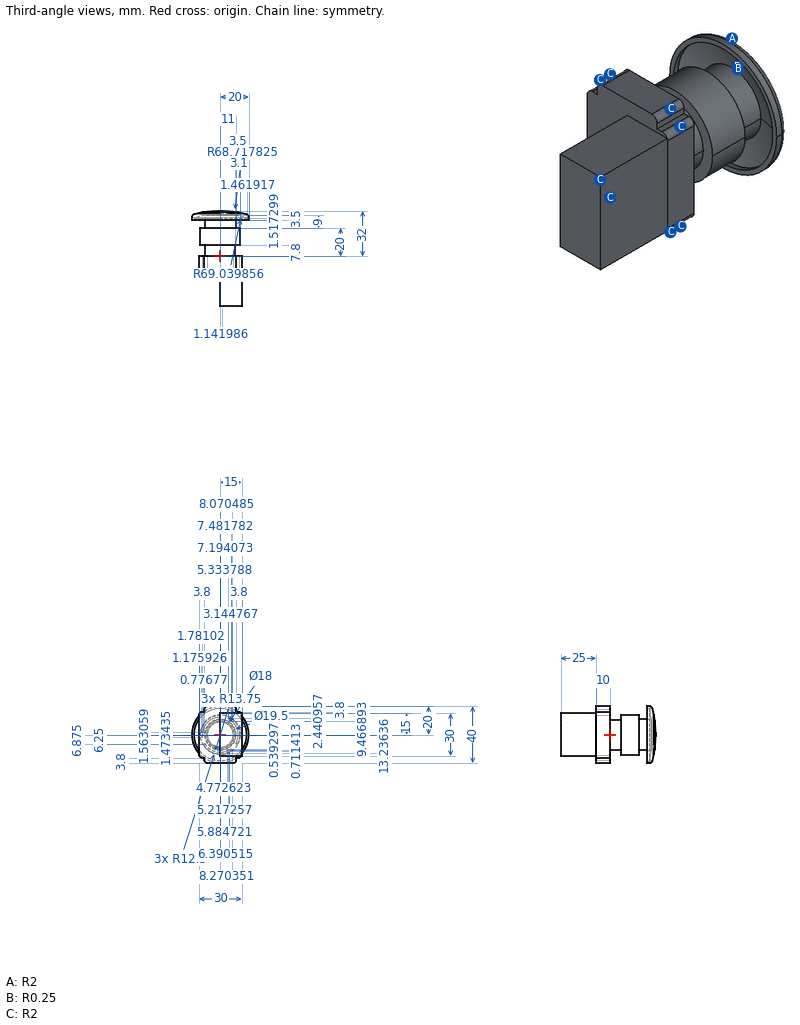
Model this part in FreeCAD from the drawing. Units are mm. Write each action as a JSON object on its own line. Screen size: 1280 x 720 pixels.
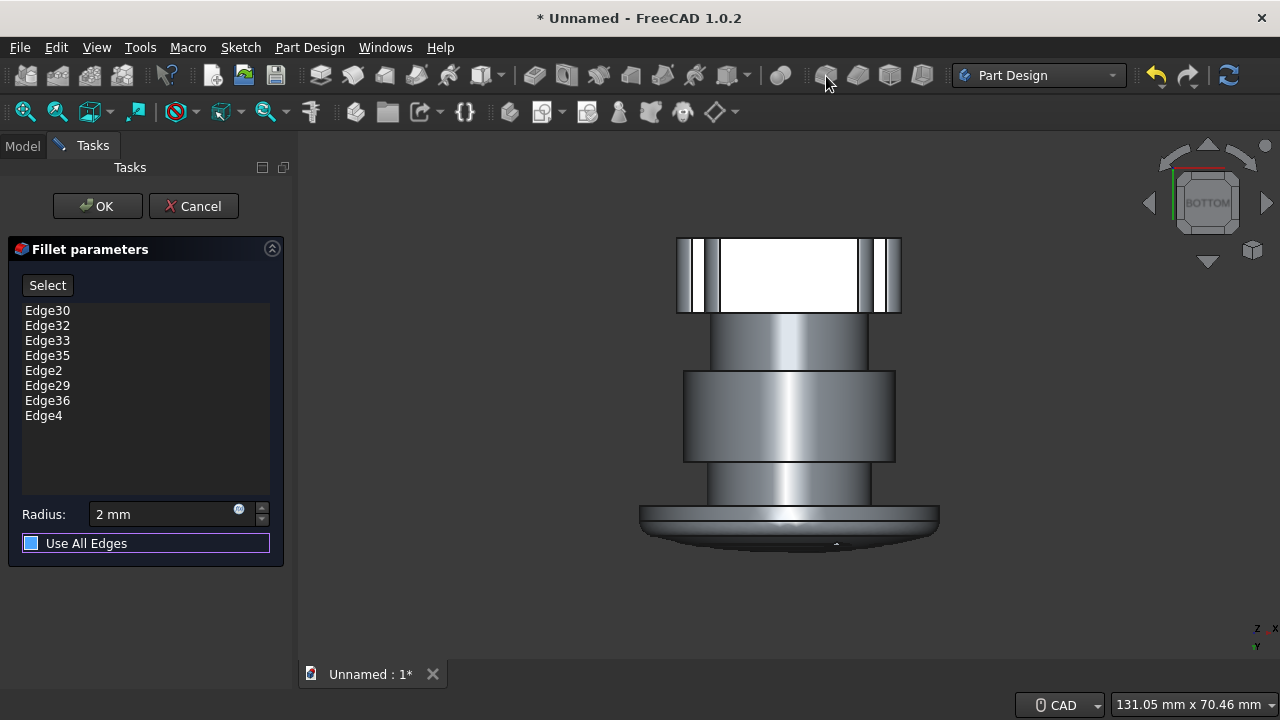
{"action": "left_click", "coordinate": [98, 206]}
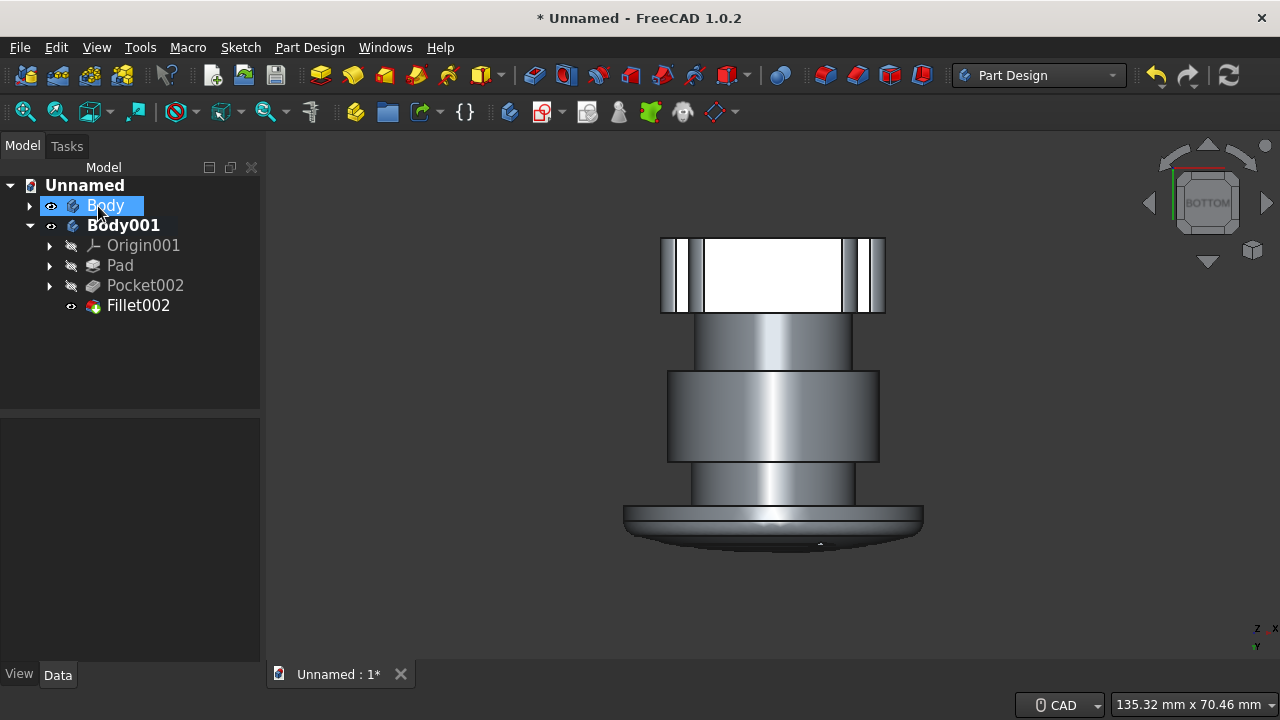
{"action": "left_click", "coordinate": [26, 112]}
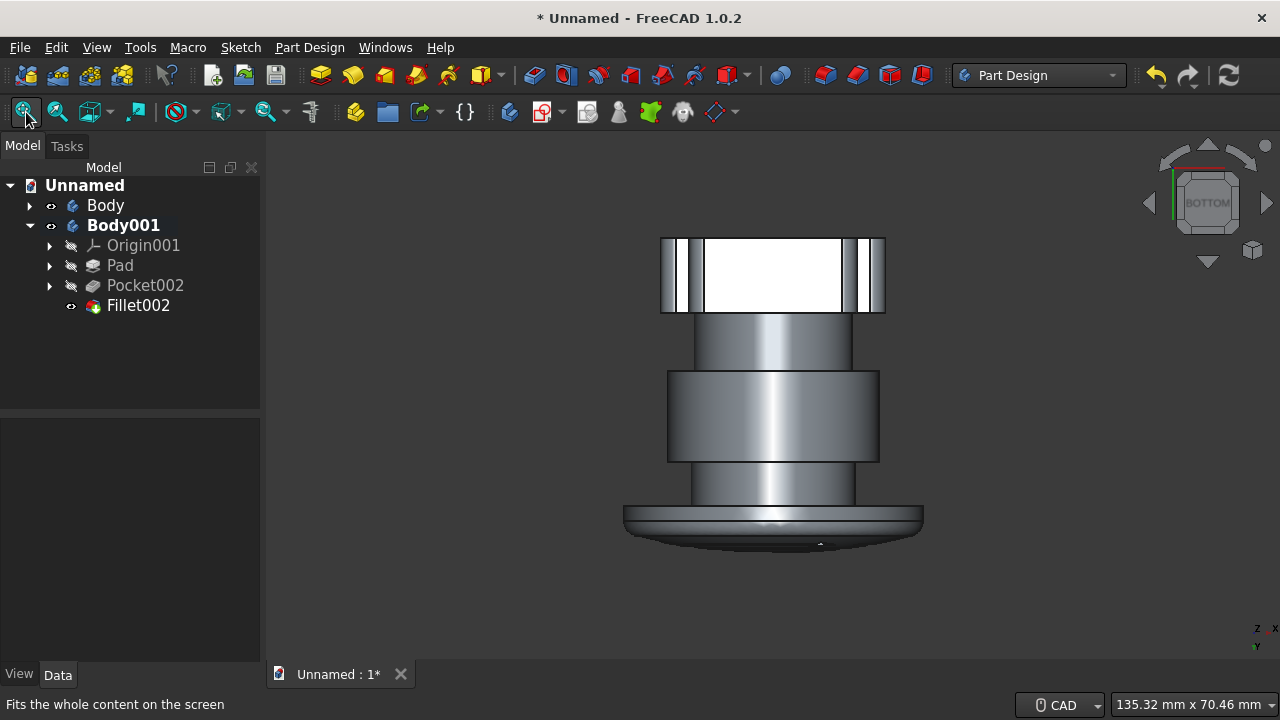
{"action": "left_click", "coordinate": [510, 112]}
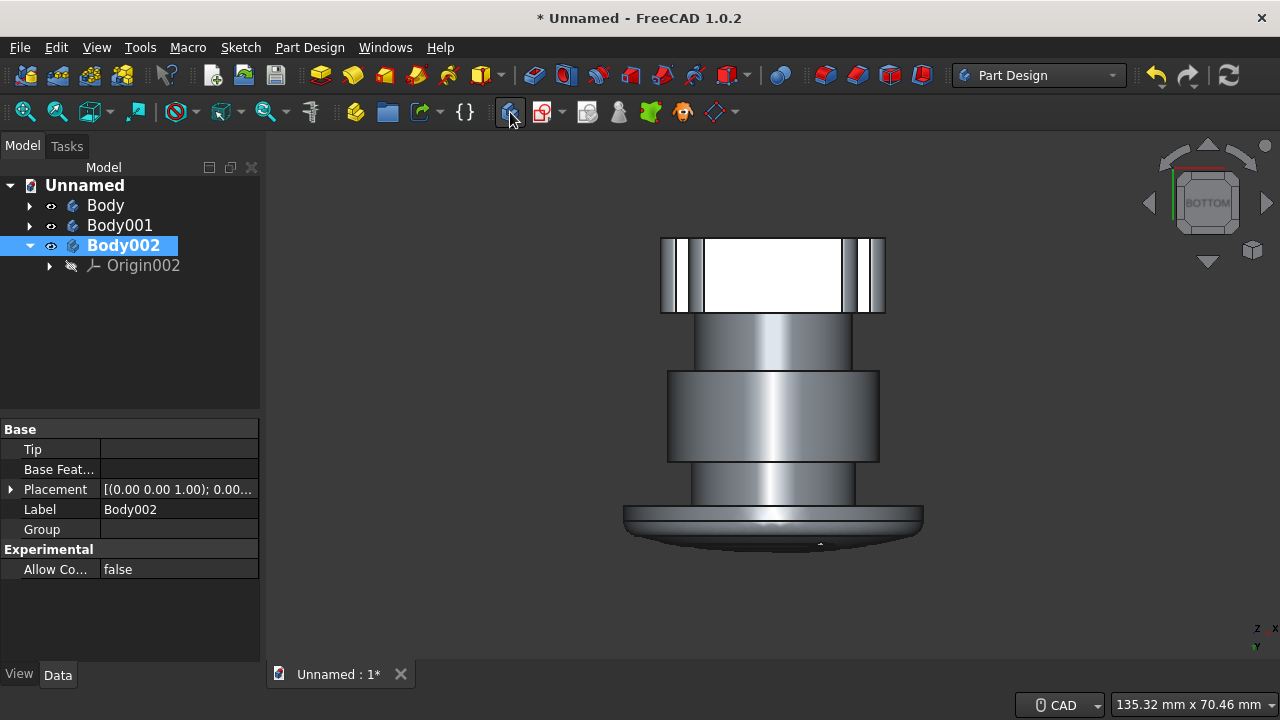
{"action": "left_click", "coordinate": [50, 266]}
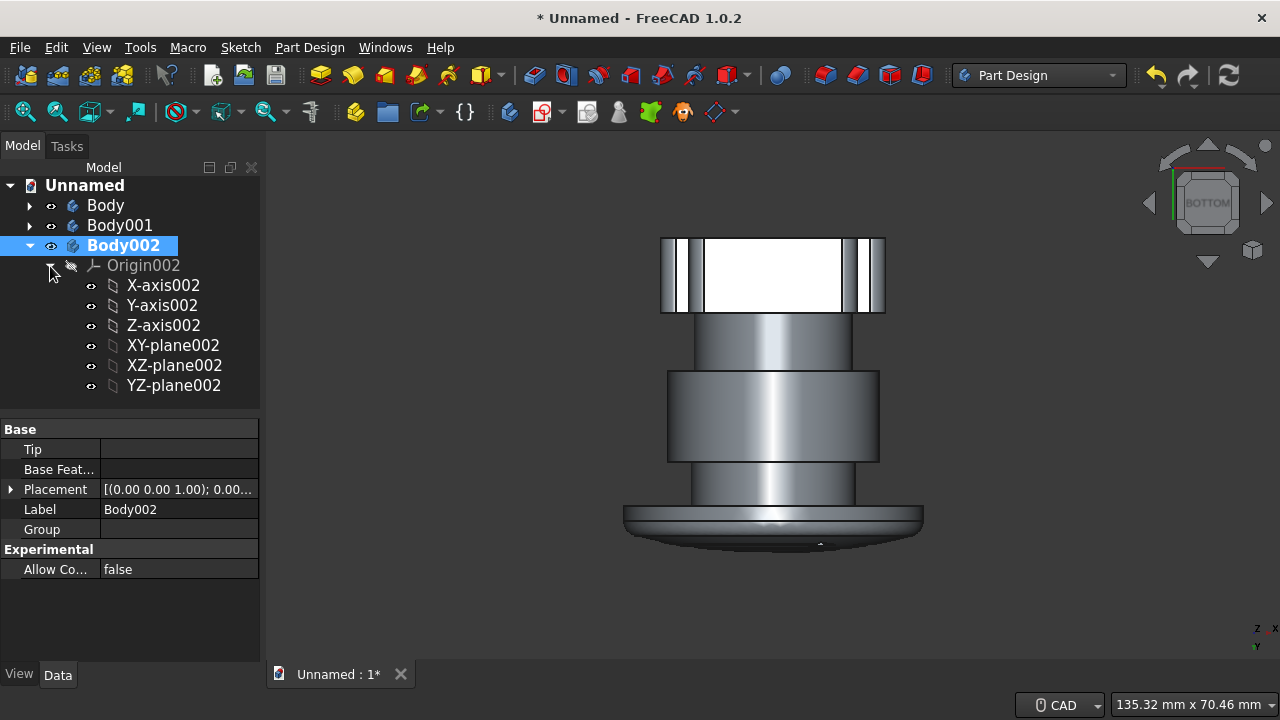
{"action": "left_click", "coordinate": [136, 366]}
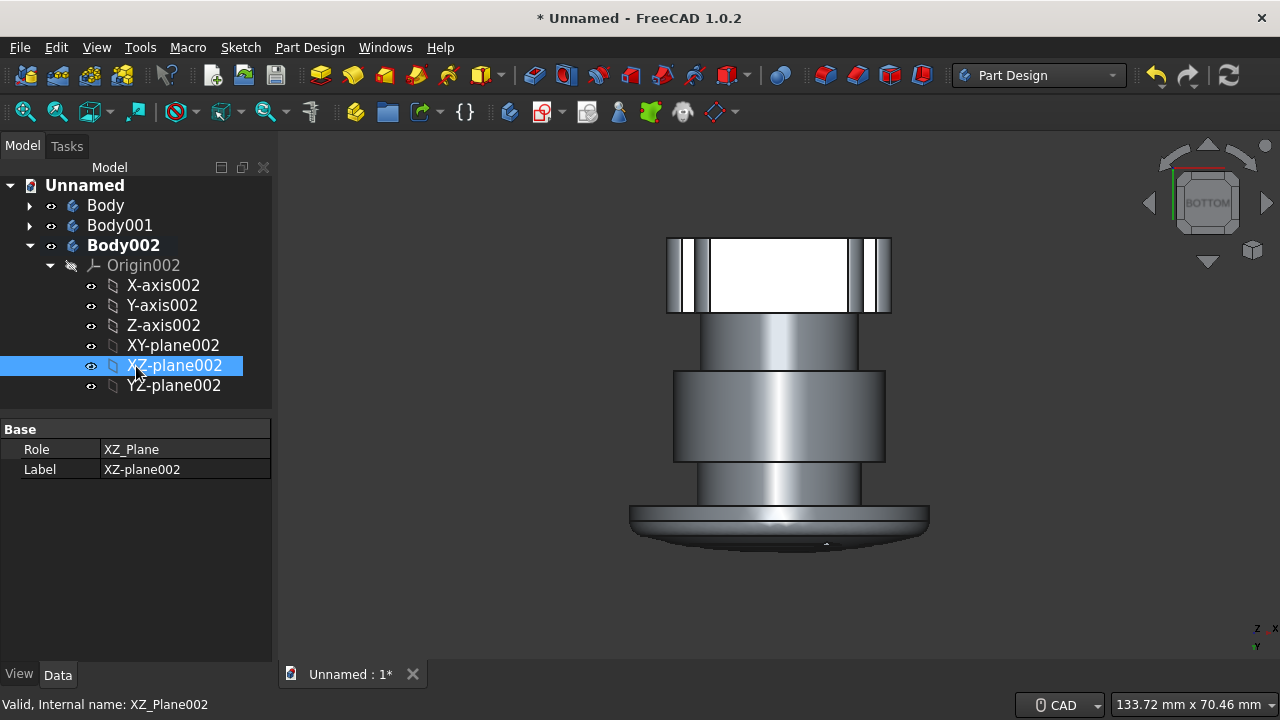
{"action": "left_click", "coordinate": [716, 112]}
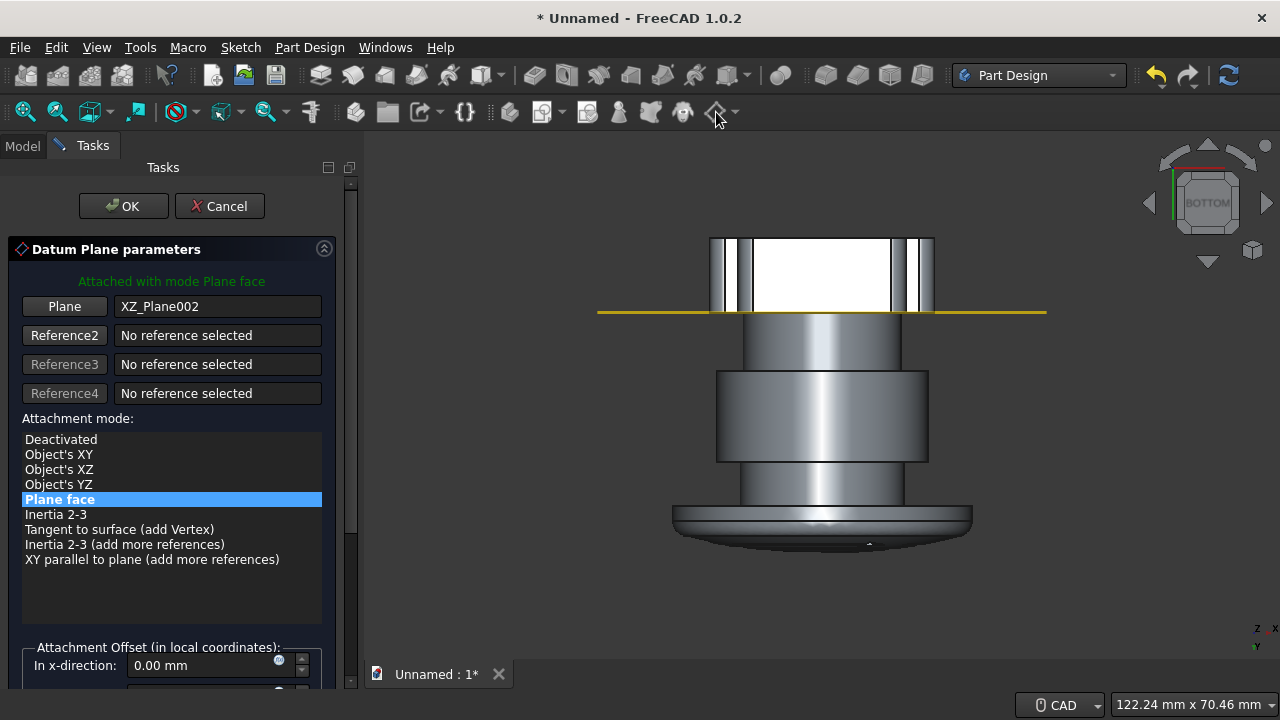
{"action": "scroll", "coordinate": [351, 432], "scroll_direction": "down", "scroll_amount": 2}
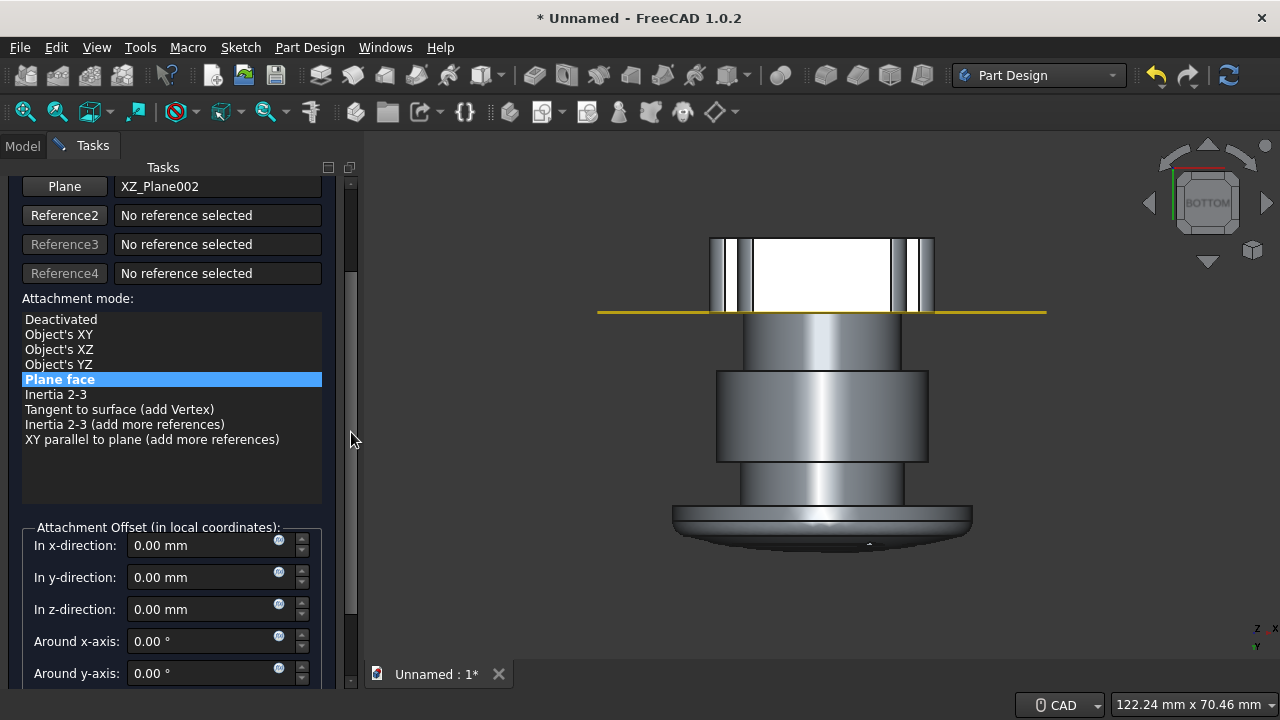
{"action": "triple_click", "coordinate": [210, 609]}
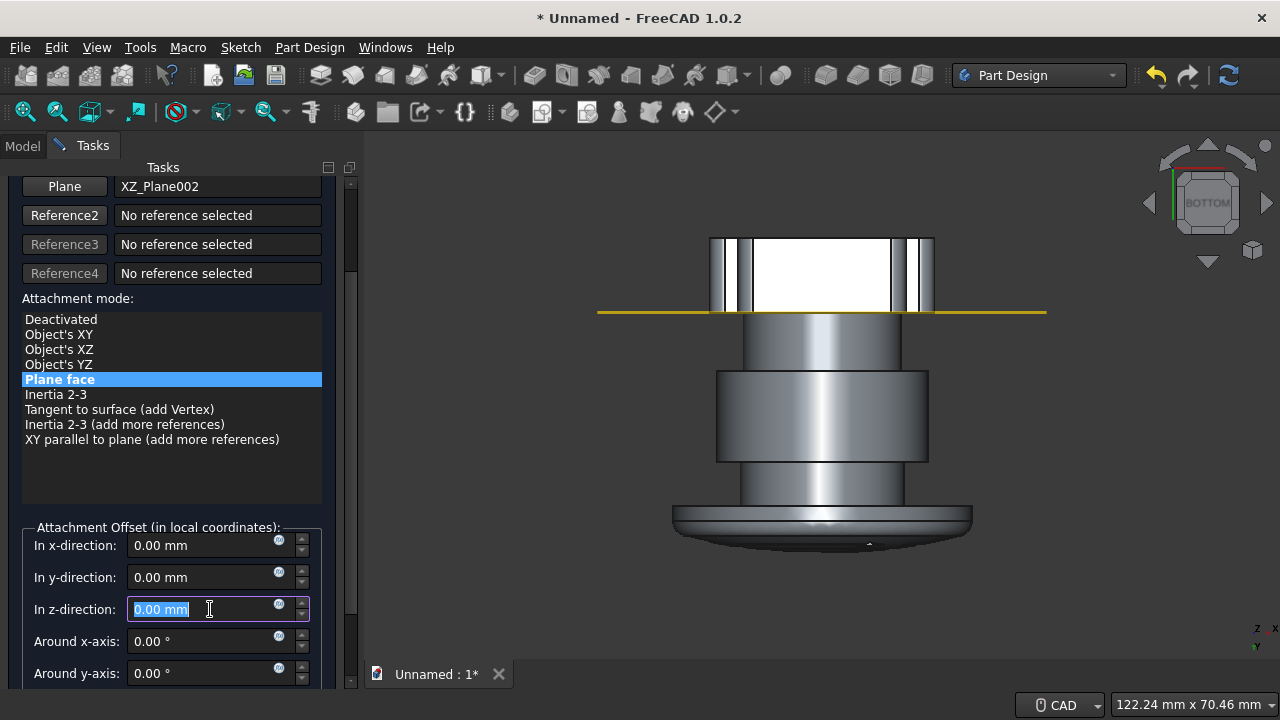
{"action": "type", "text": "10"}
{"action": "key", "text": "Tab"}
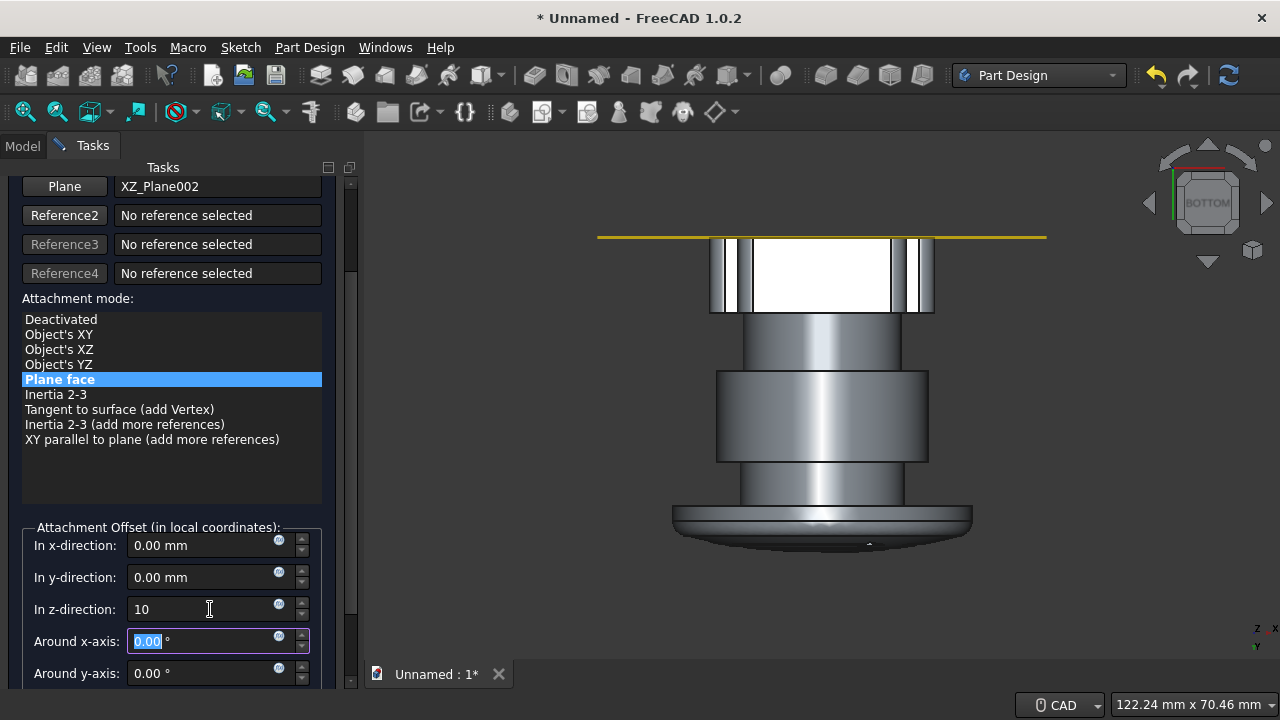
{"action": "scroll", "coordinate": [351, 432], "scroll_direction": "up", "scroll_amount": 3}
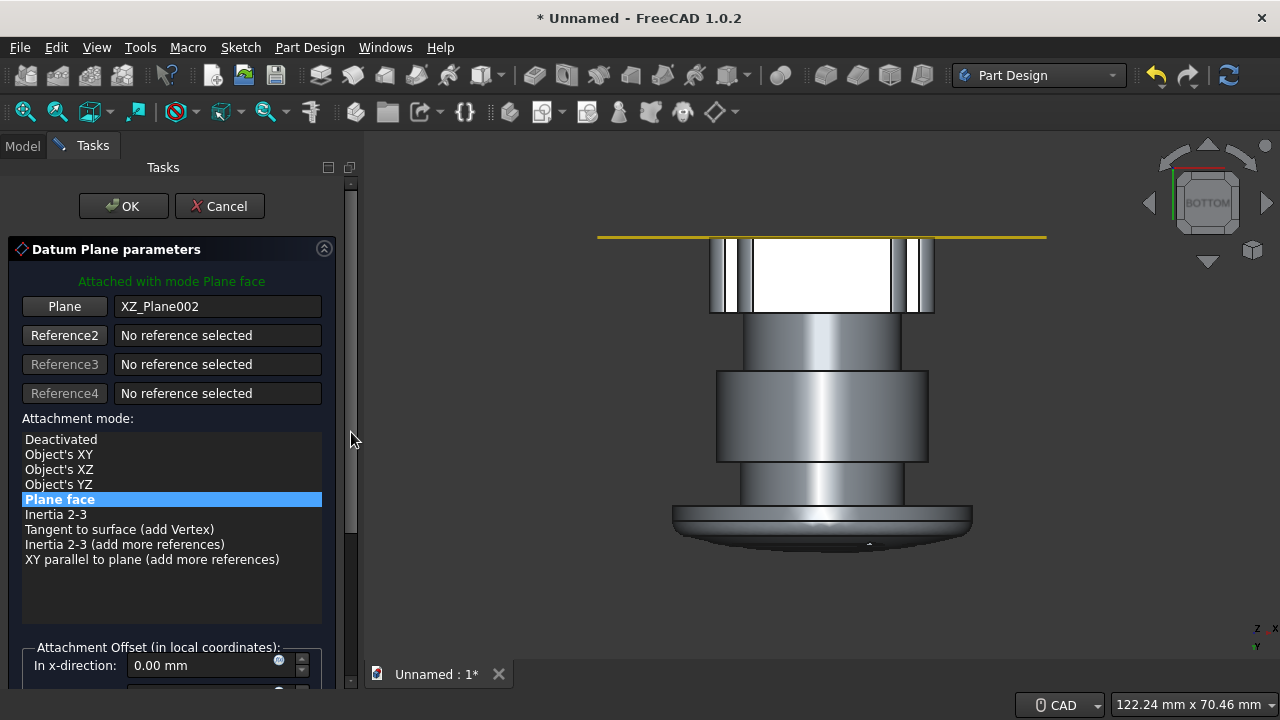
{"action": "left_click", "coordinate": [124, 206]}